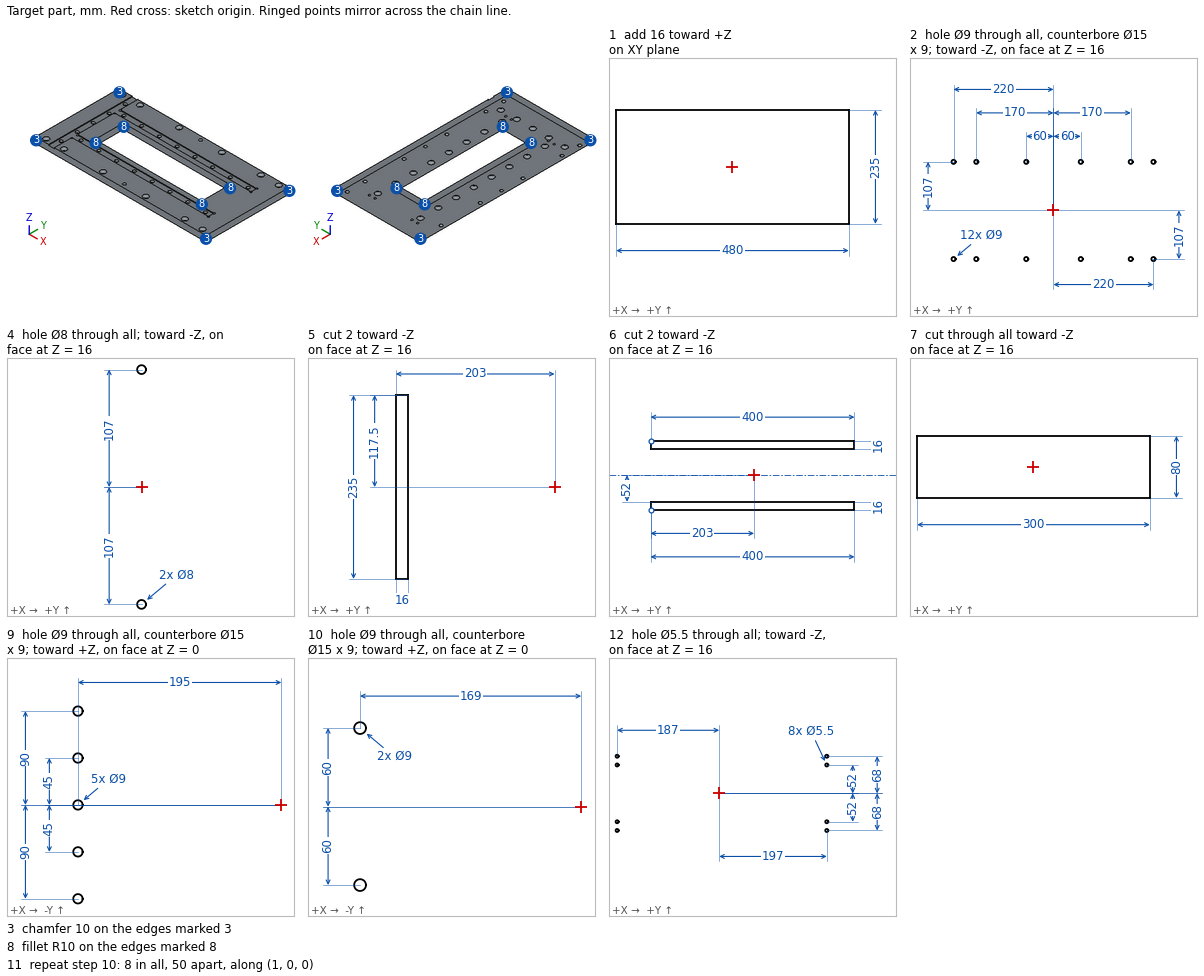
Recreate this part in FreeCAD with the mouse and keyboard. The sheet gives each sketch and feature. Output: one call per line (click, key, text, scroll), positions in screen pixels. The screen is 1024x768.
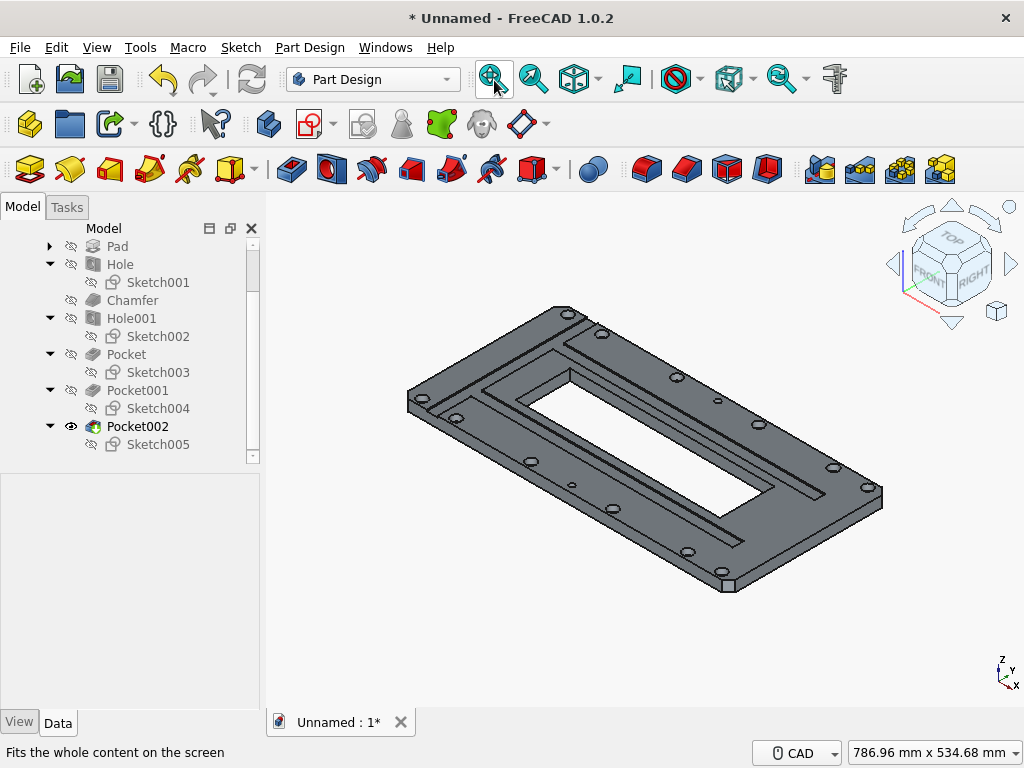
scroll(774, 492, up, 5)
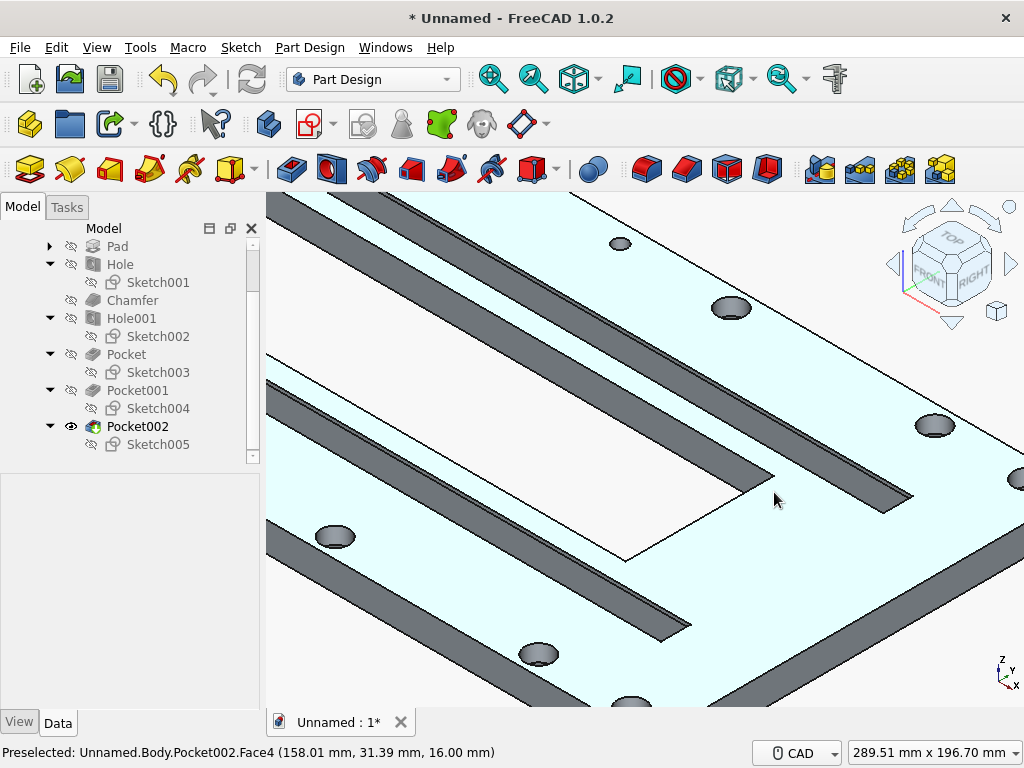
click(494, 80)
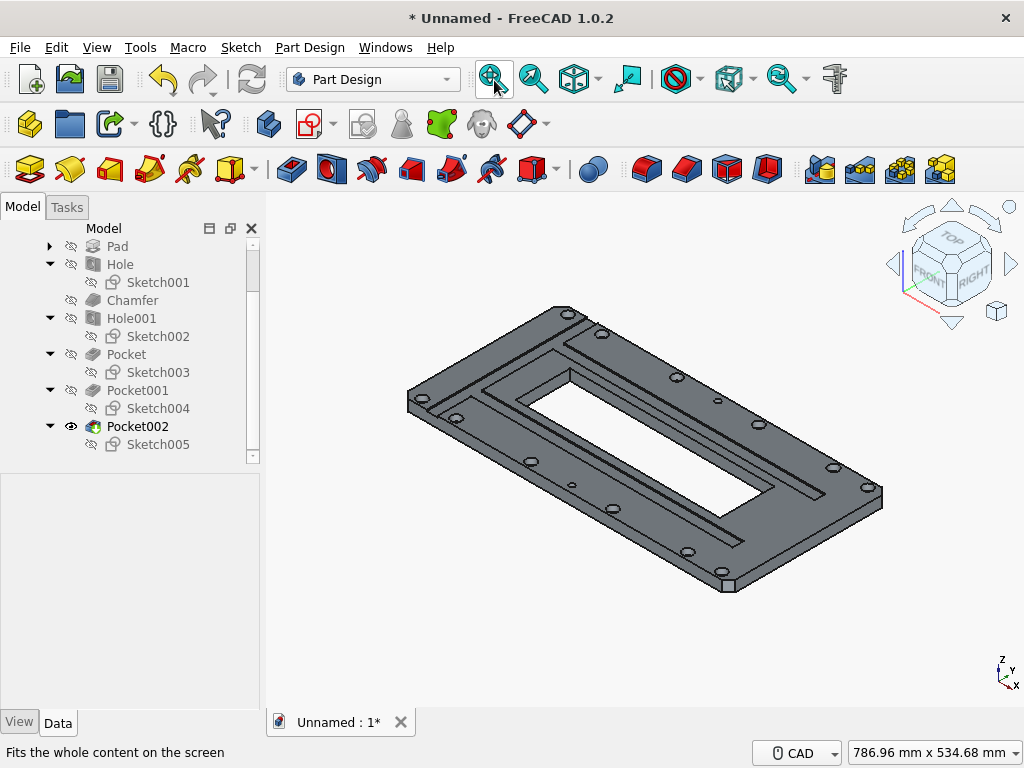
key(1)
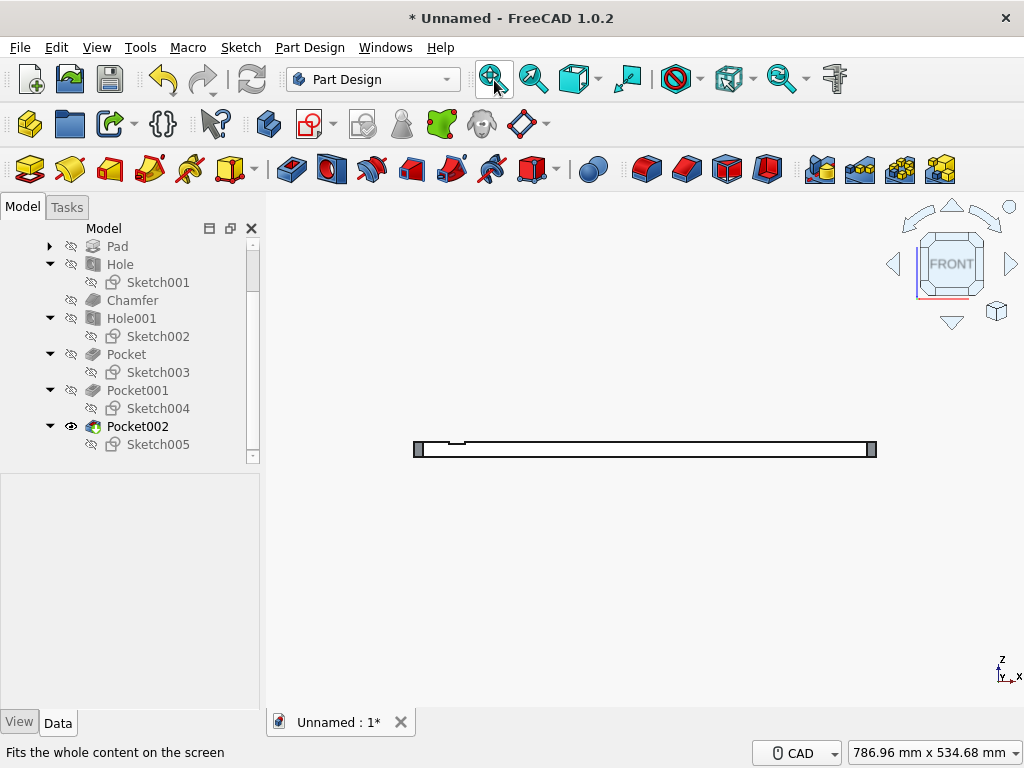
scroll(789, 449, up, 5)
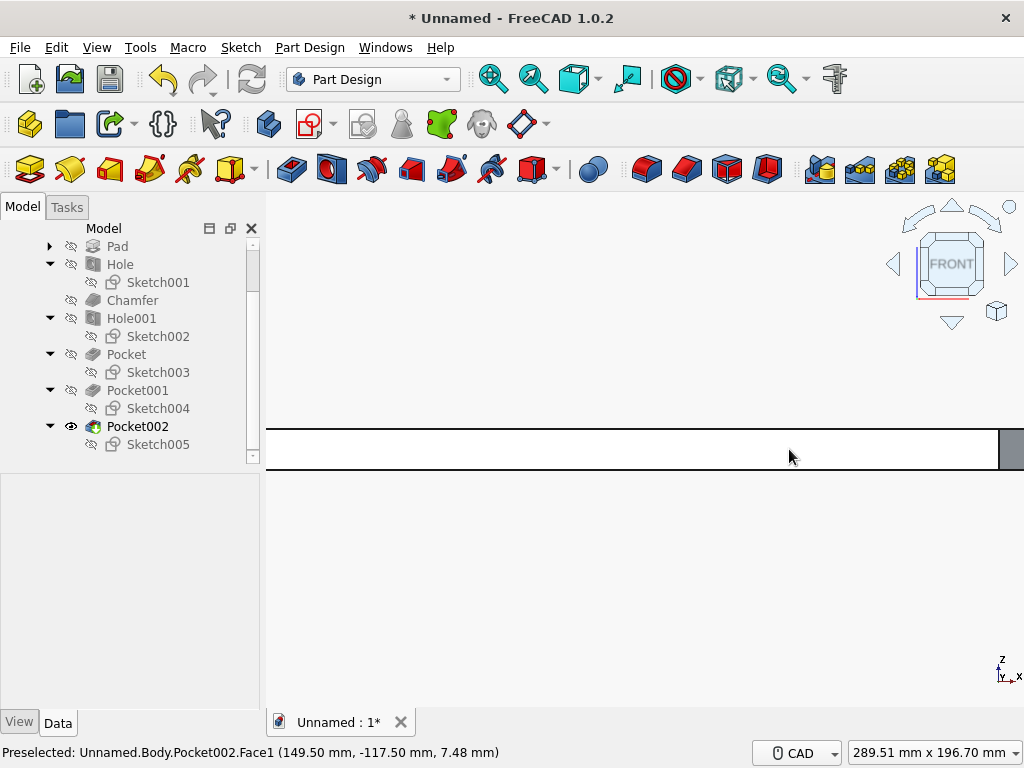
click(494, 80)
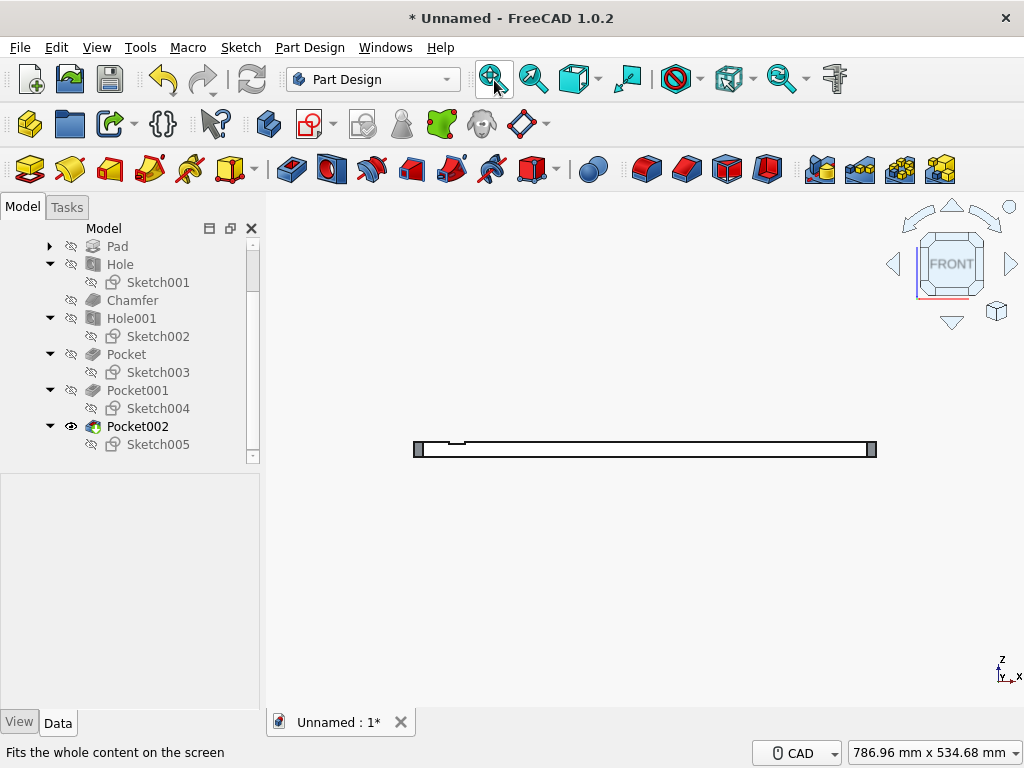
key(3)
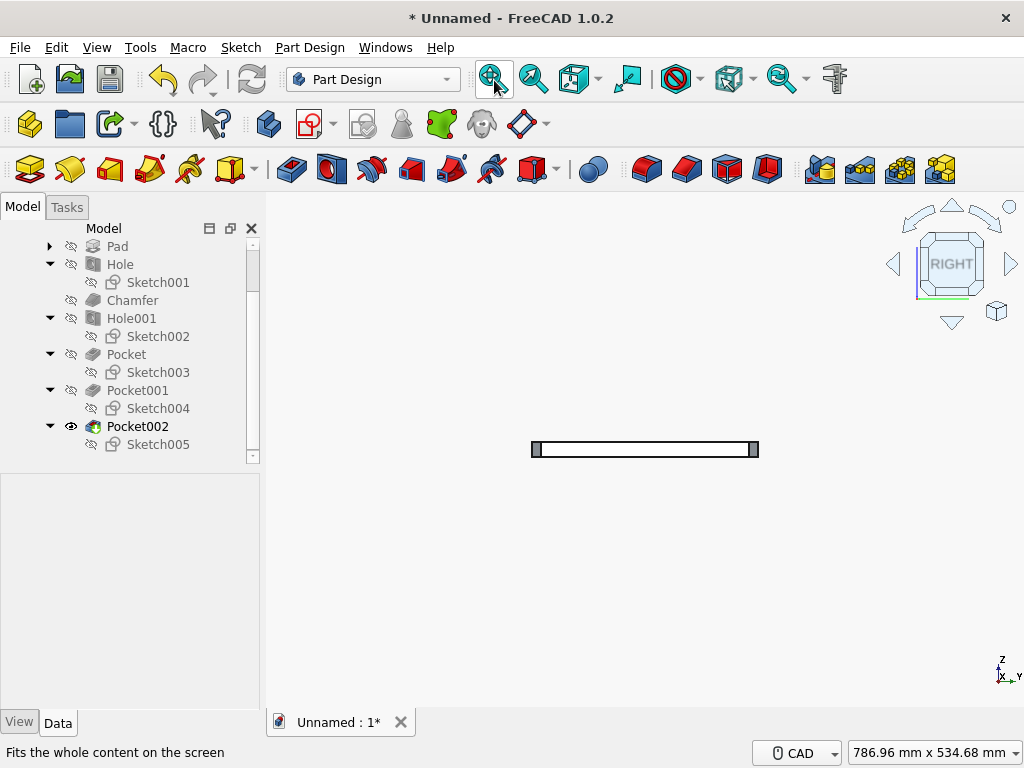
click(494, 80)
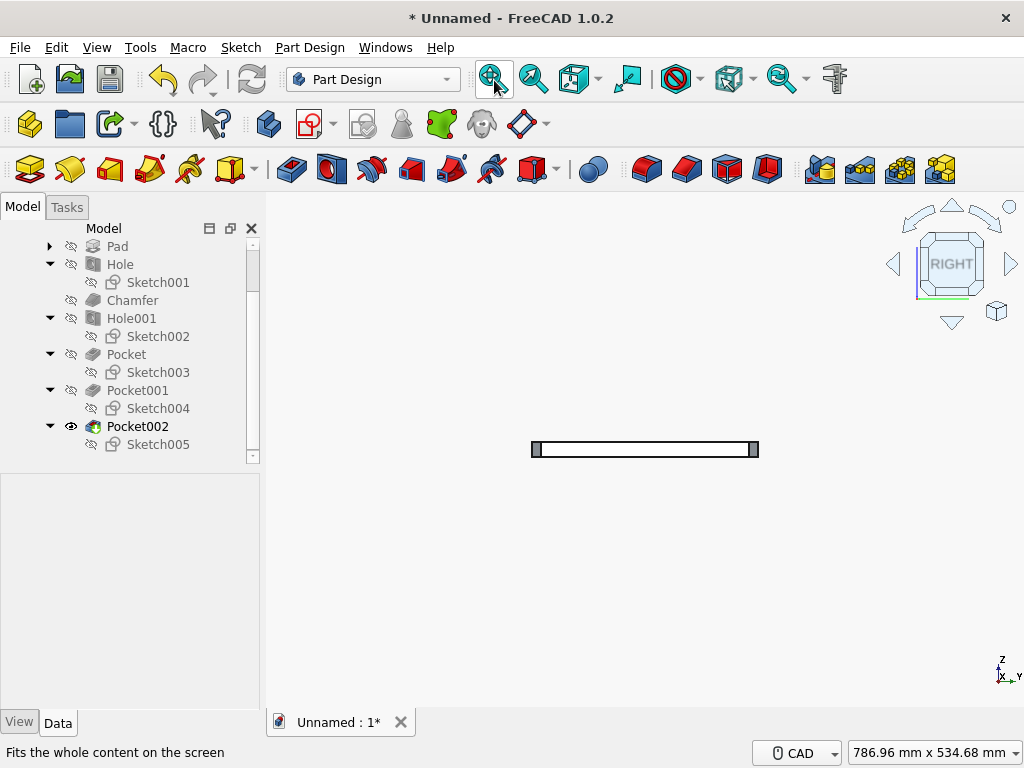
scroll(684, 448, up, 5)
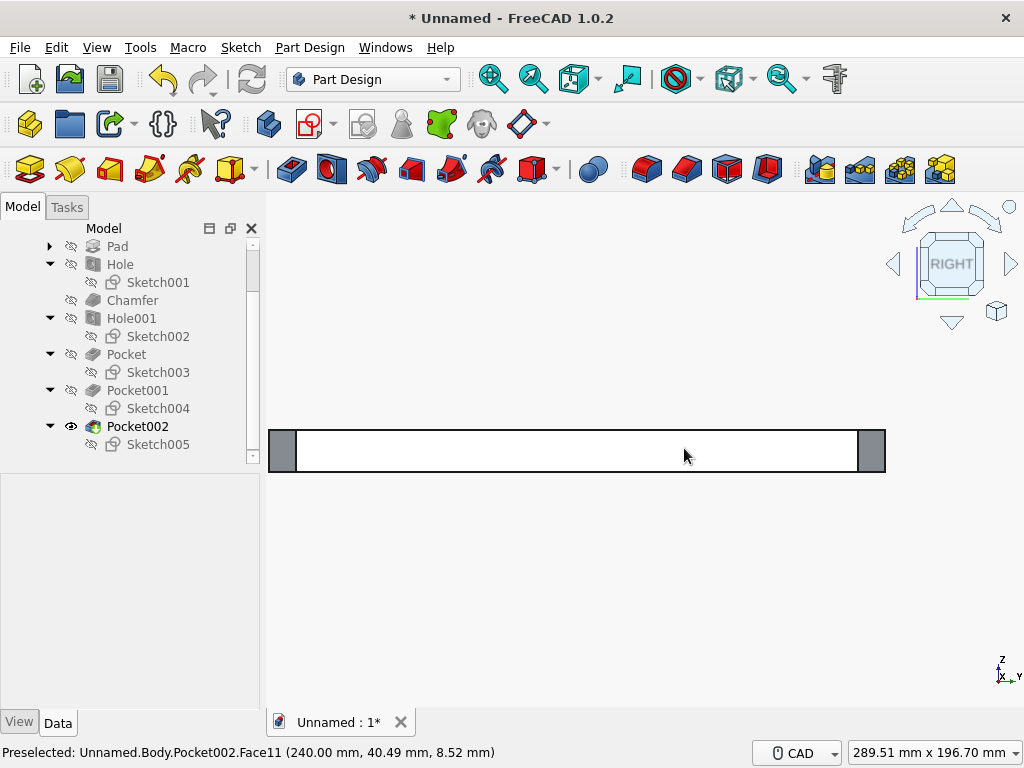
click(494, 80)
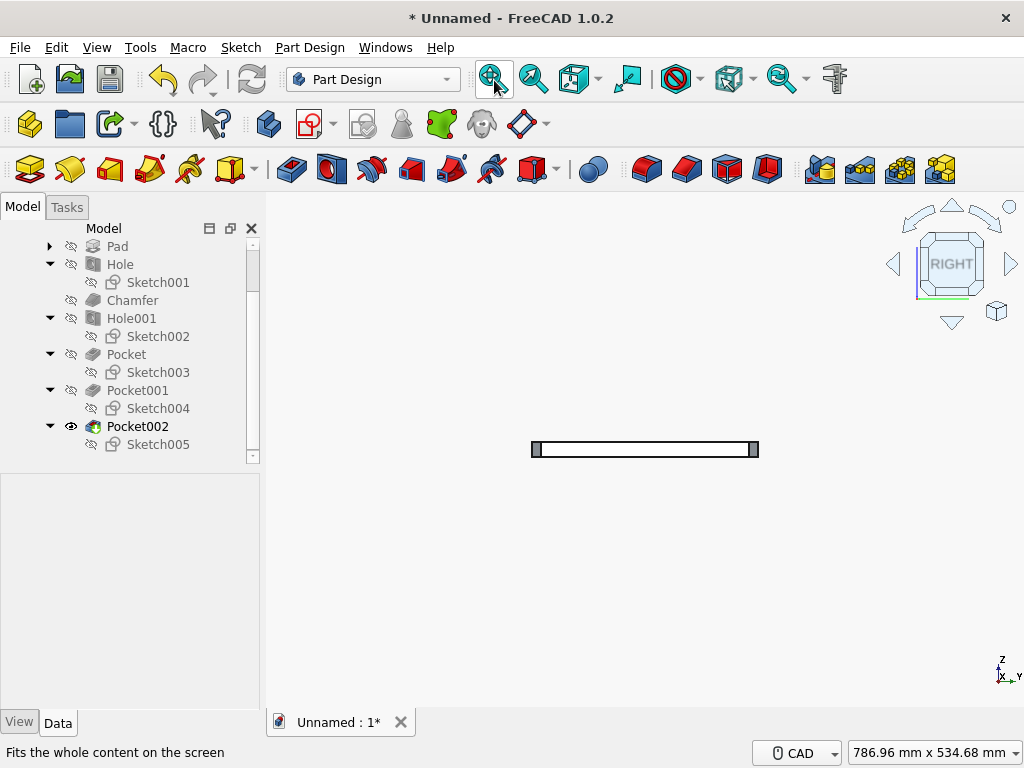
key(5)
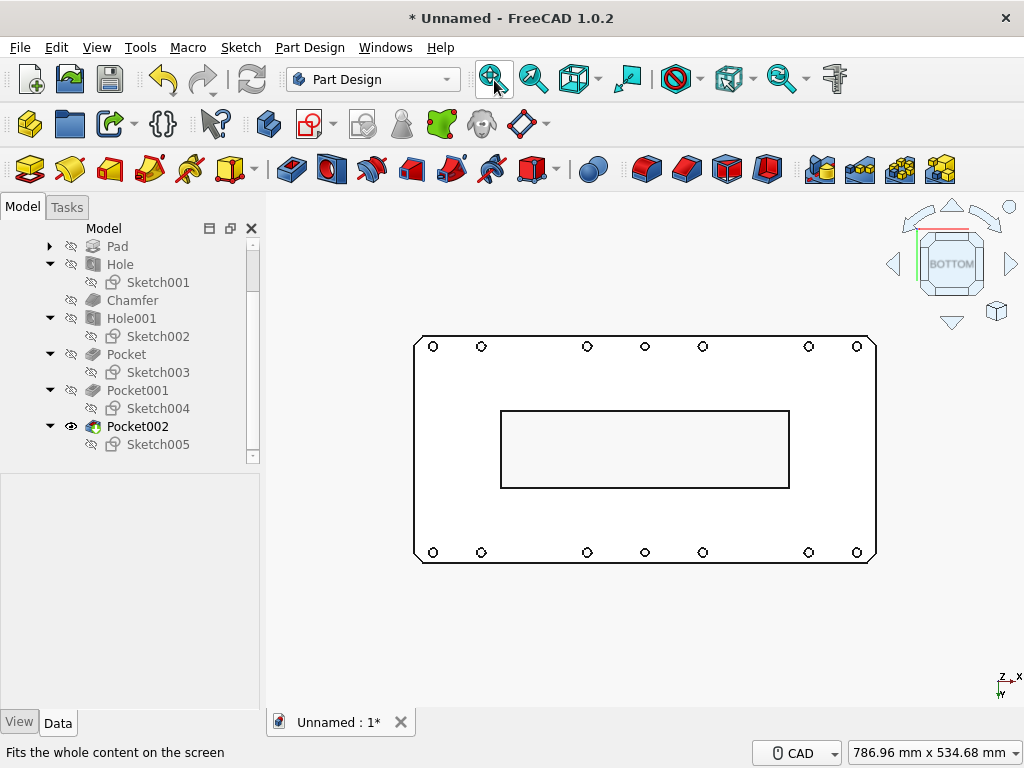
scroll(789, 487, up, 5)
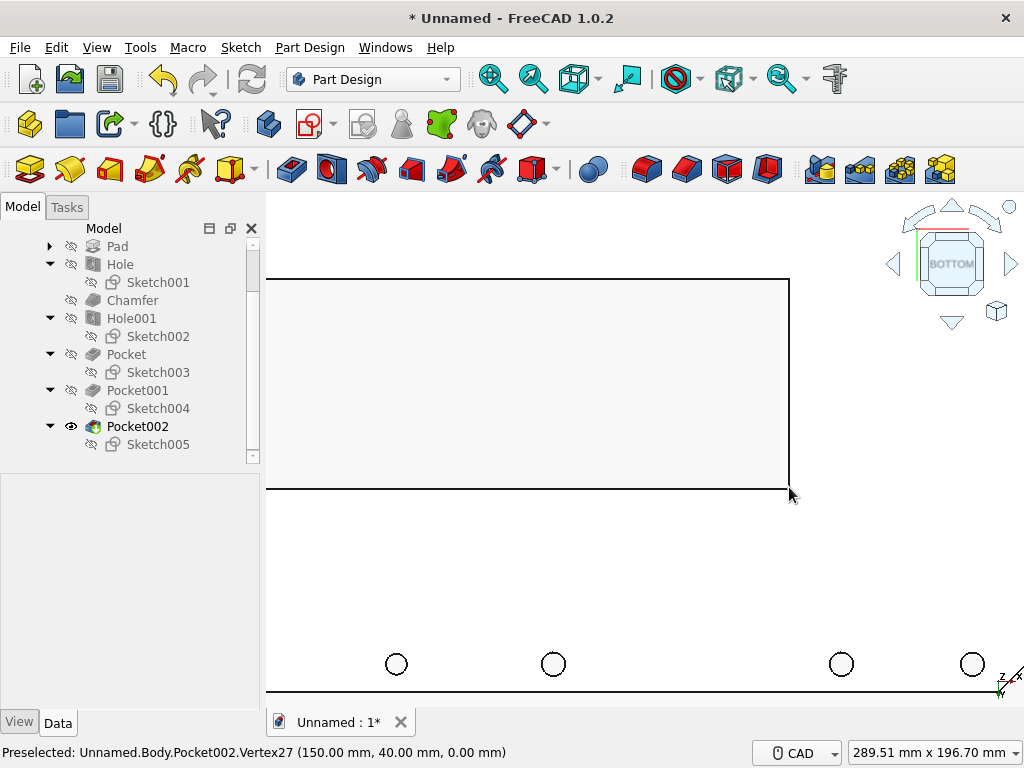
click(494, 80)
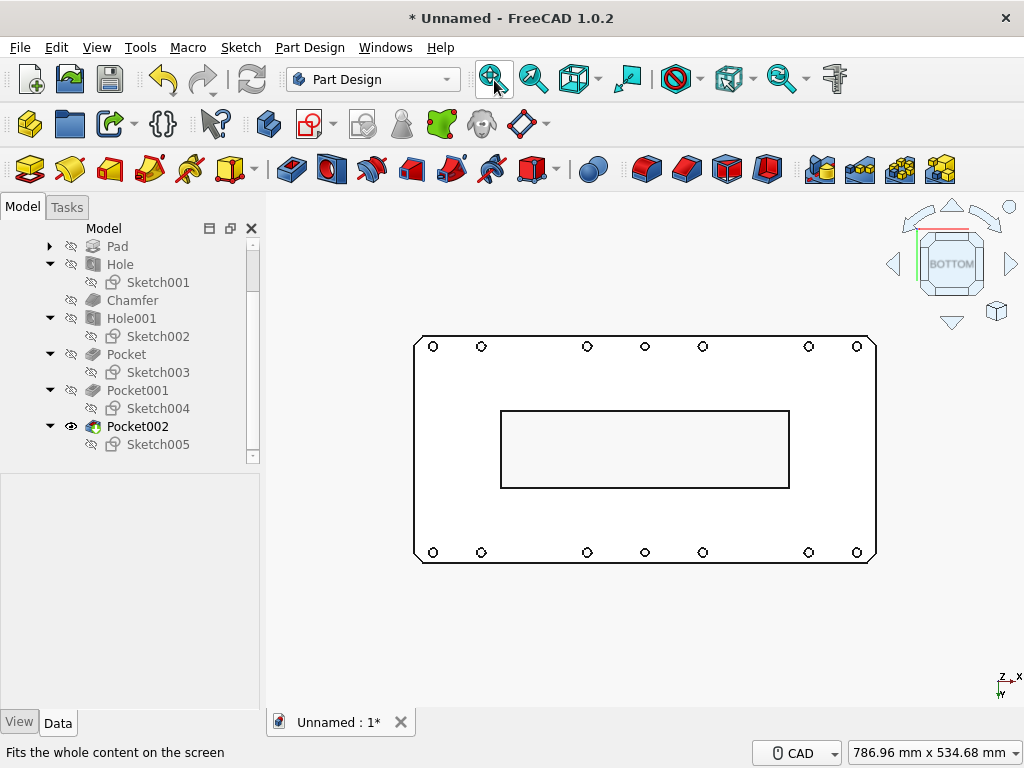
key(4)